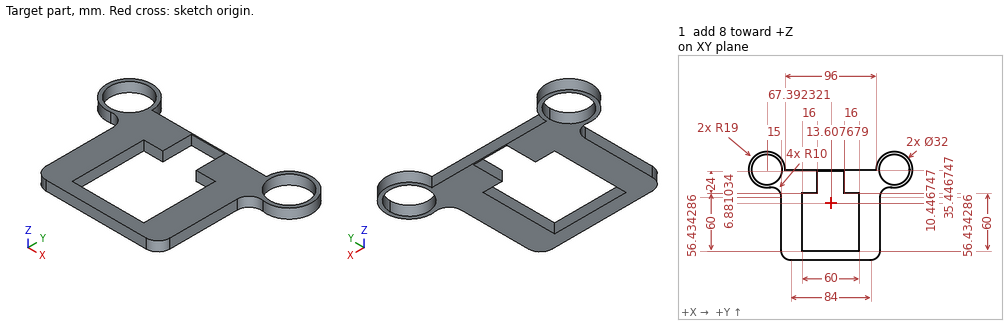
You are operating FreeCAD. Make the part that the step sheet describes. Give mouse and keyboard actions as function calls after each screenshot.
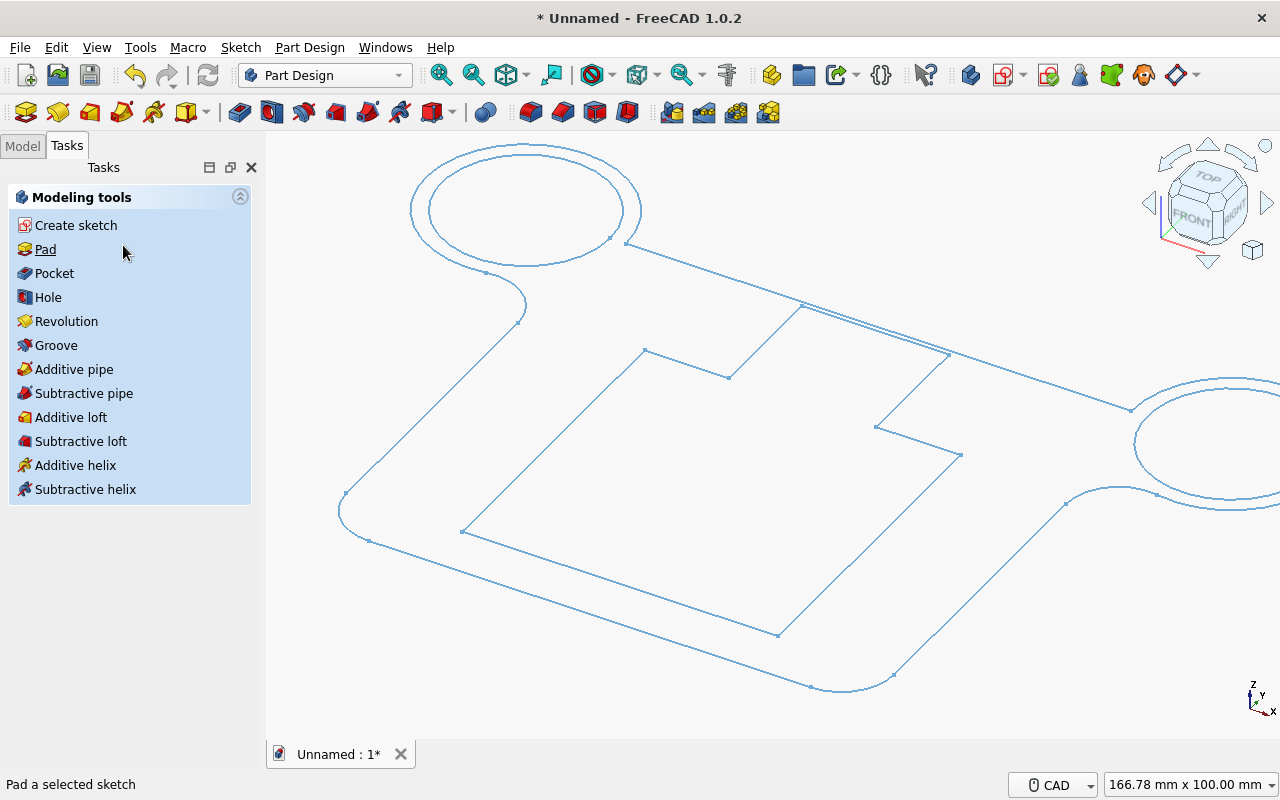
click(26, 112)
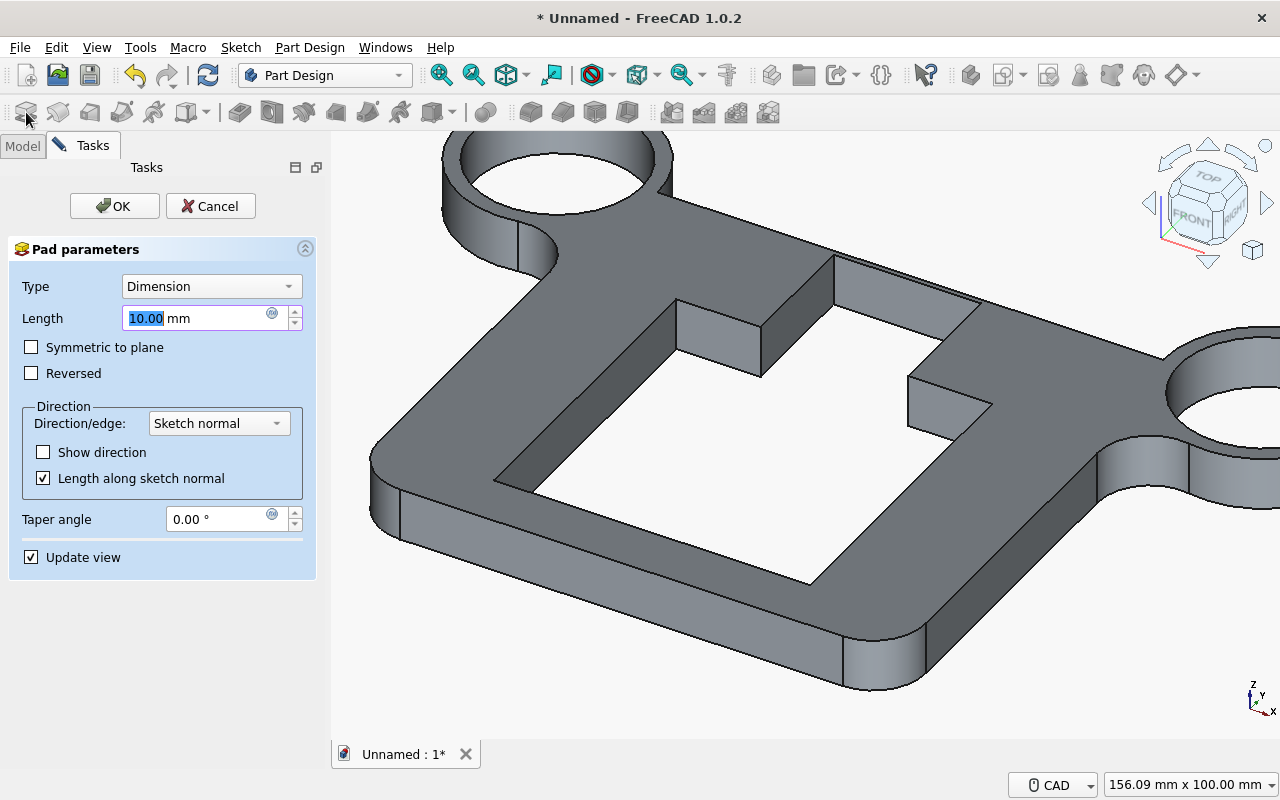
text(8)
key(Tab)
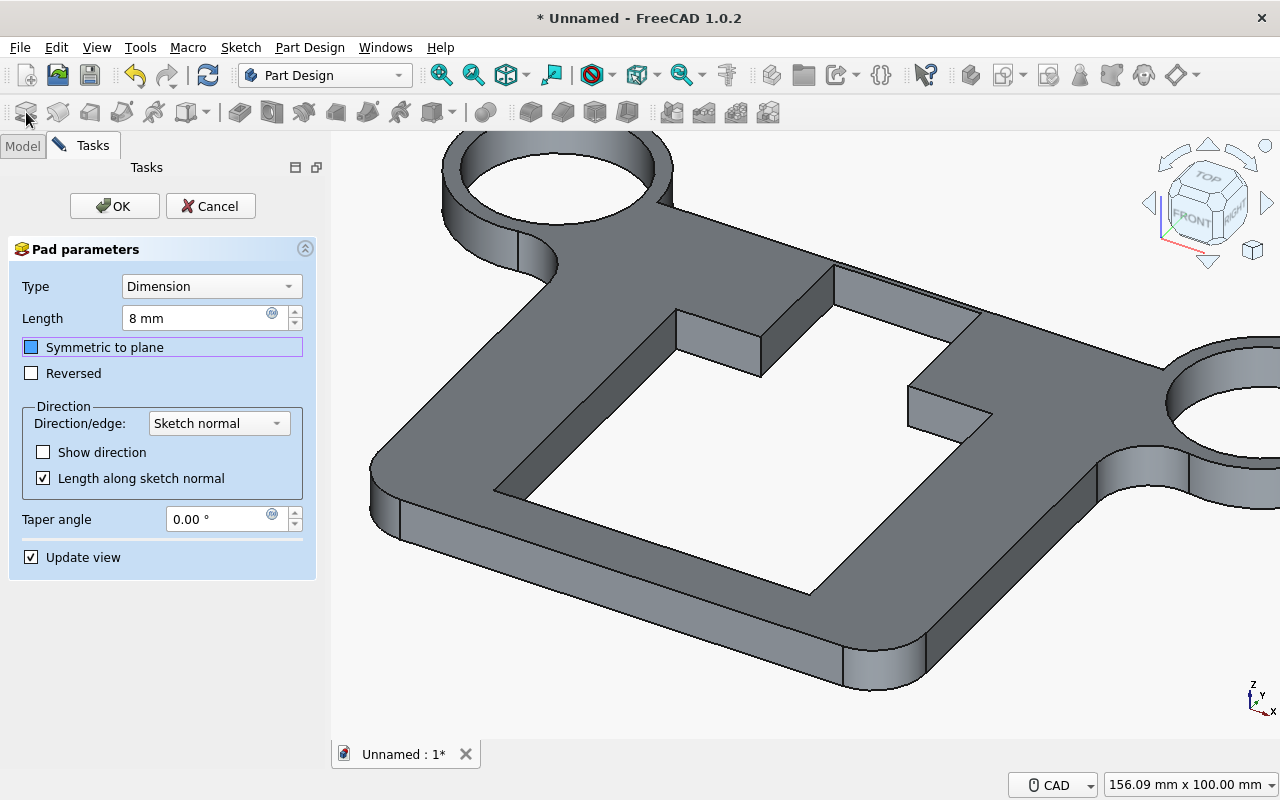
click(115, 206)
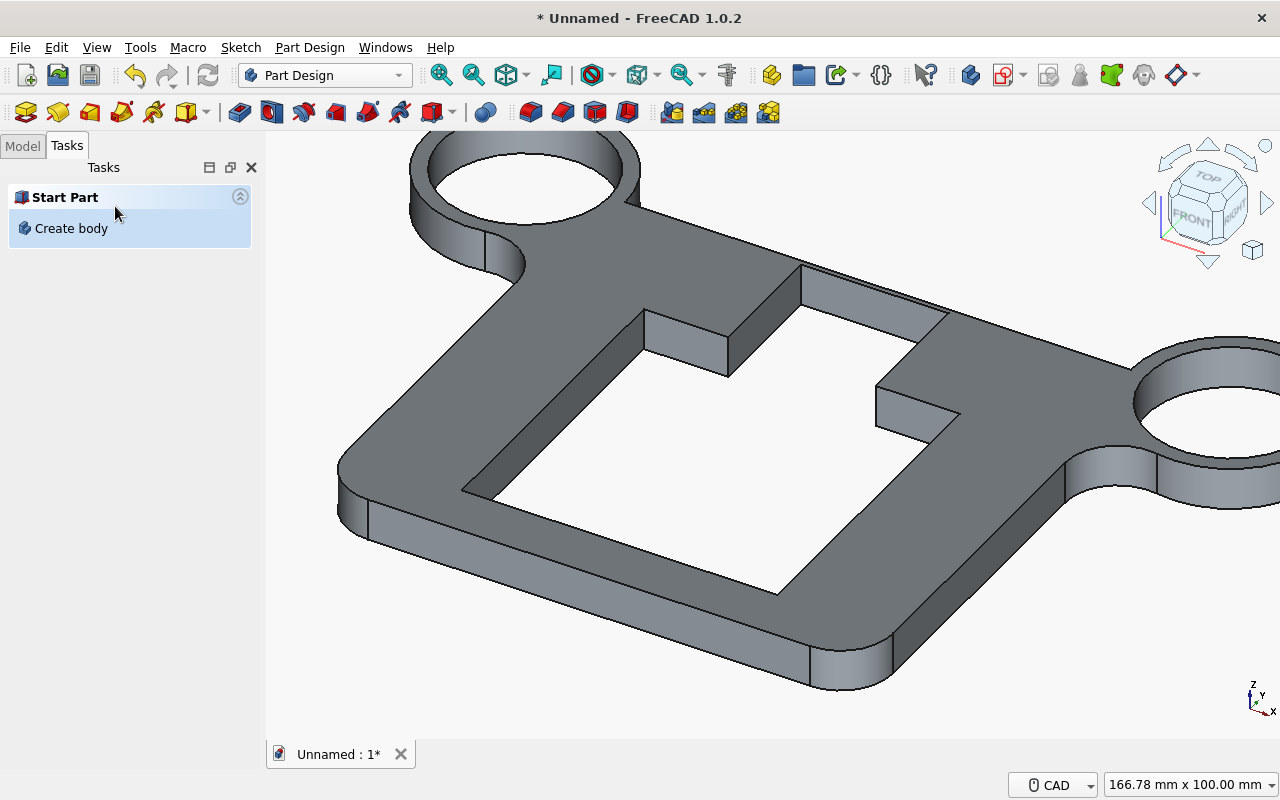
key(0)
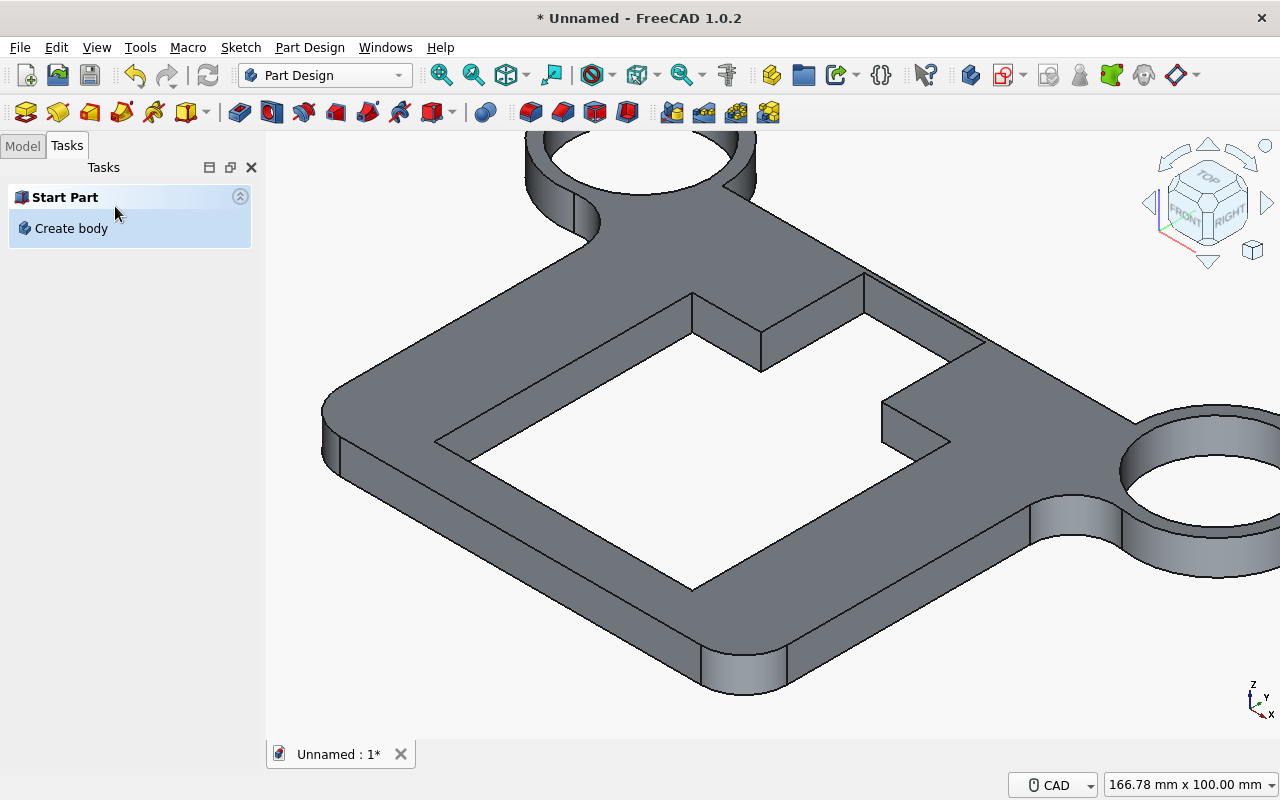
click(442, 76)